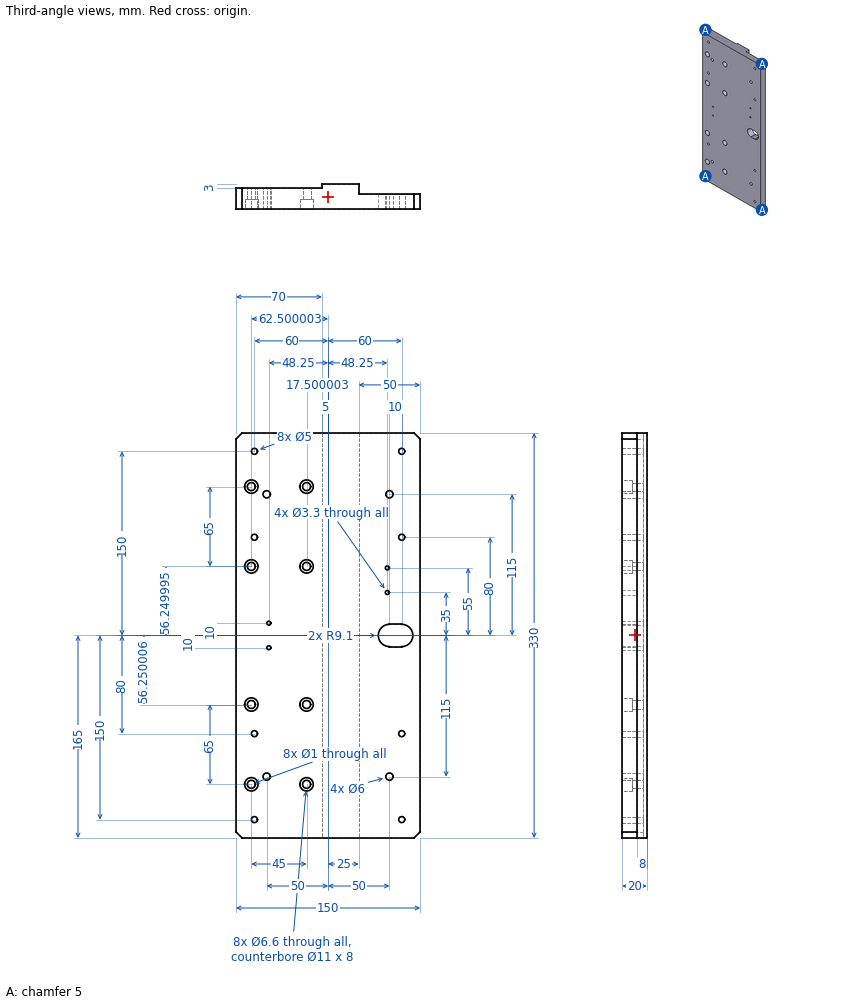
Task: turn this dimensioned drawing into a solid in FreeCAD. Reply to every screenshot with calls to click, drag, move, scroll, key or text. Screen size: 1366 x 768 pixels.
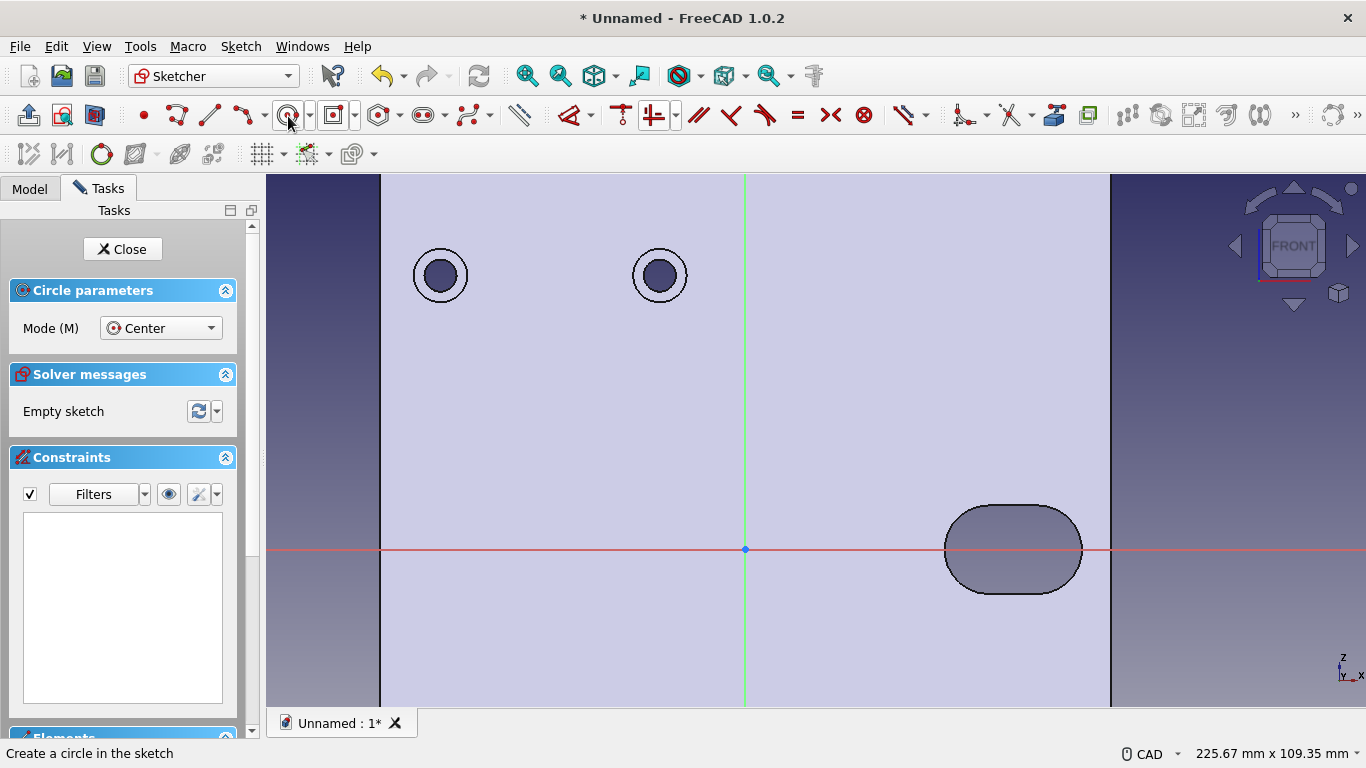
scroll(980, 379, up, 6)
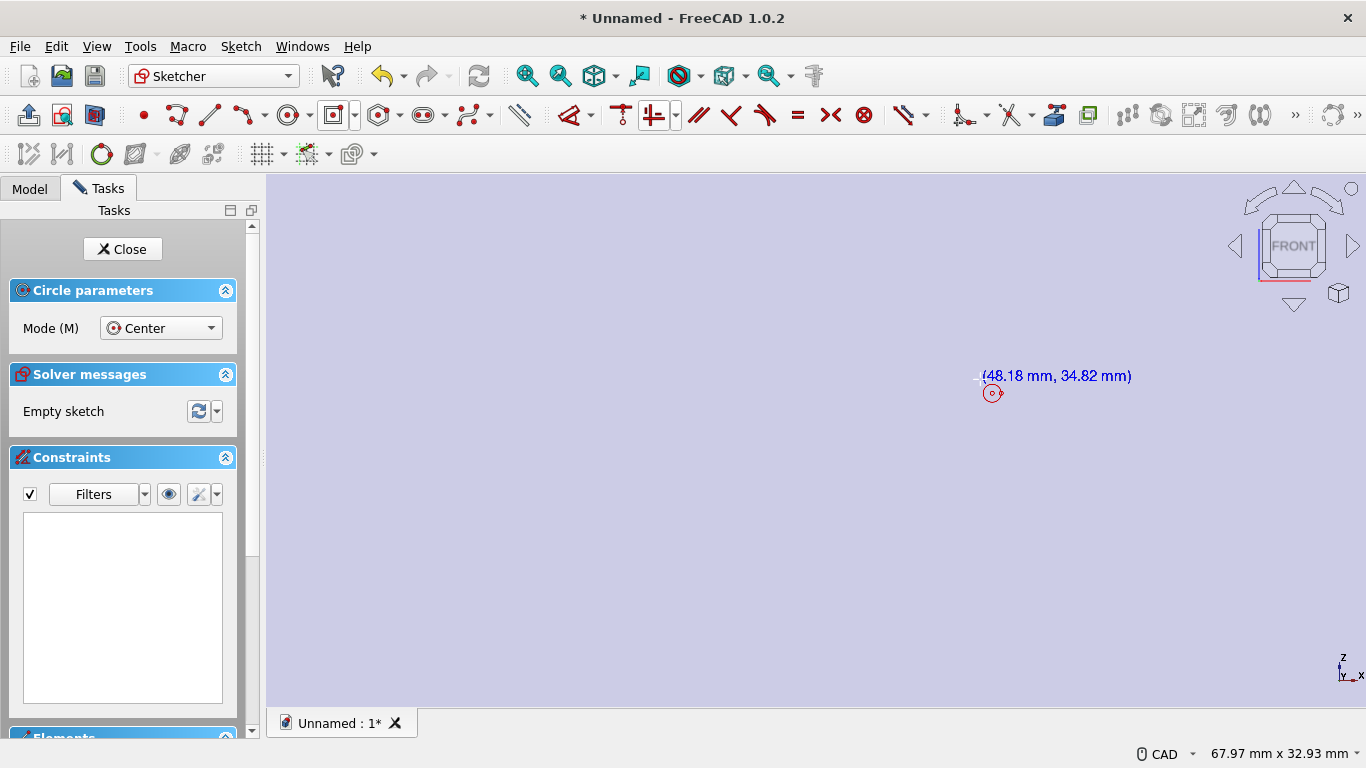
click(980, 379)
move(999, 360)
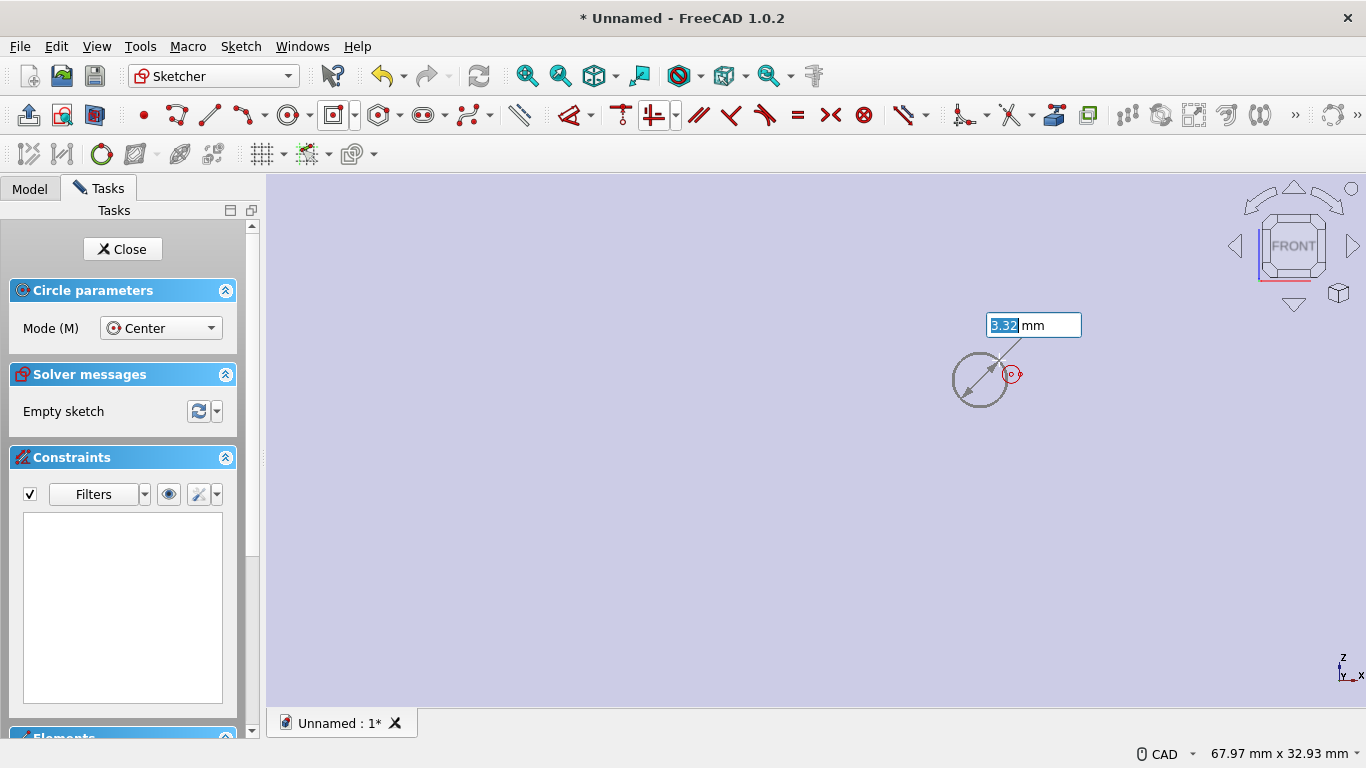
text(3.3)
key(Return)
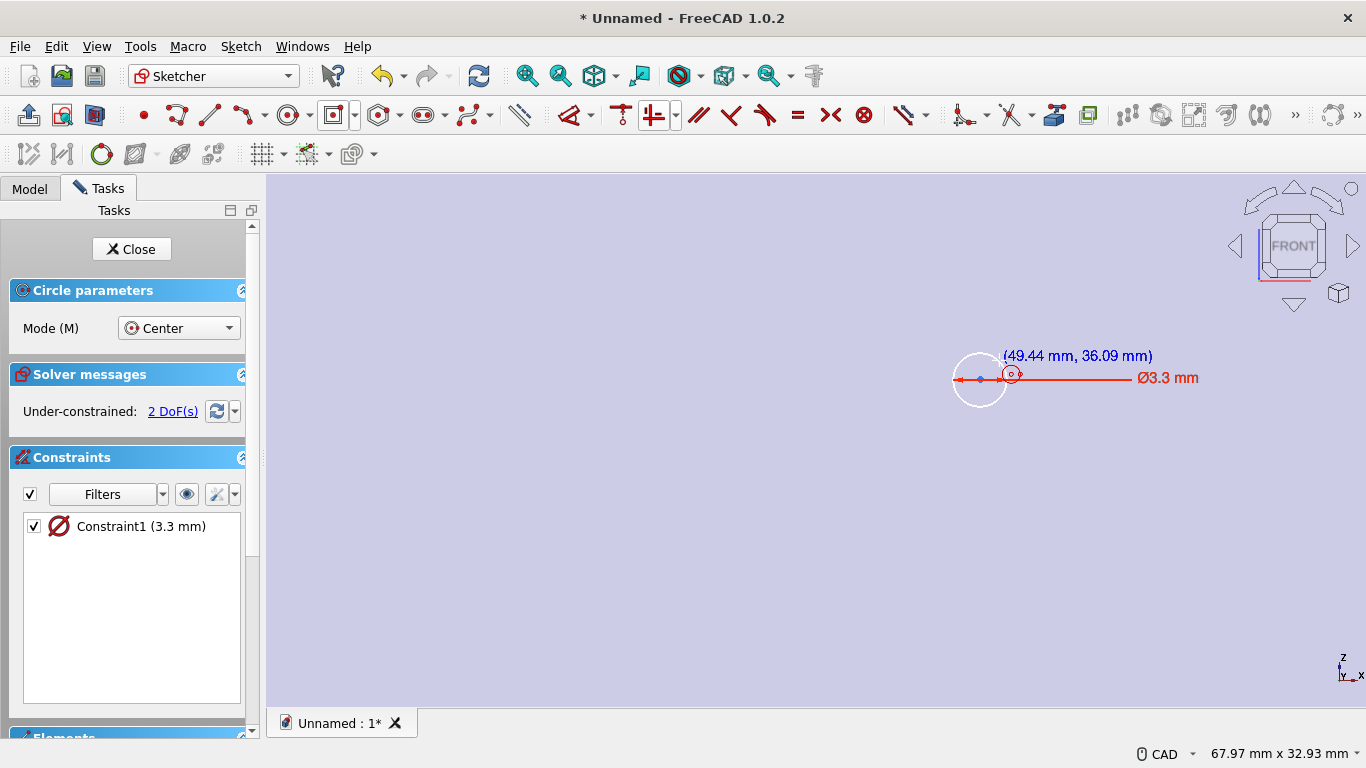
scroll(984, 380, down, 6)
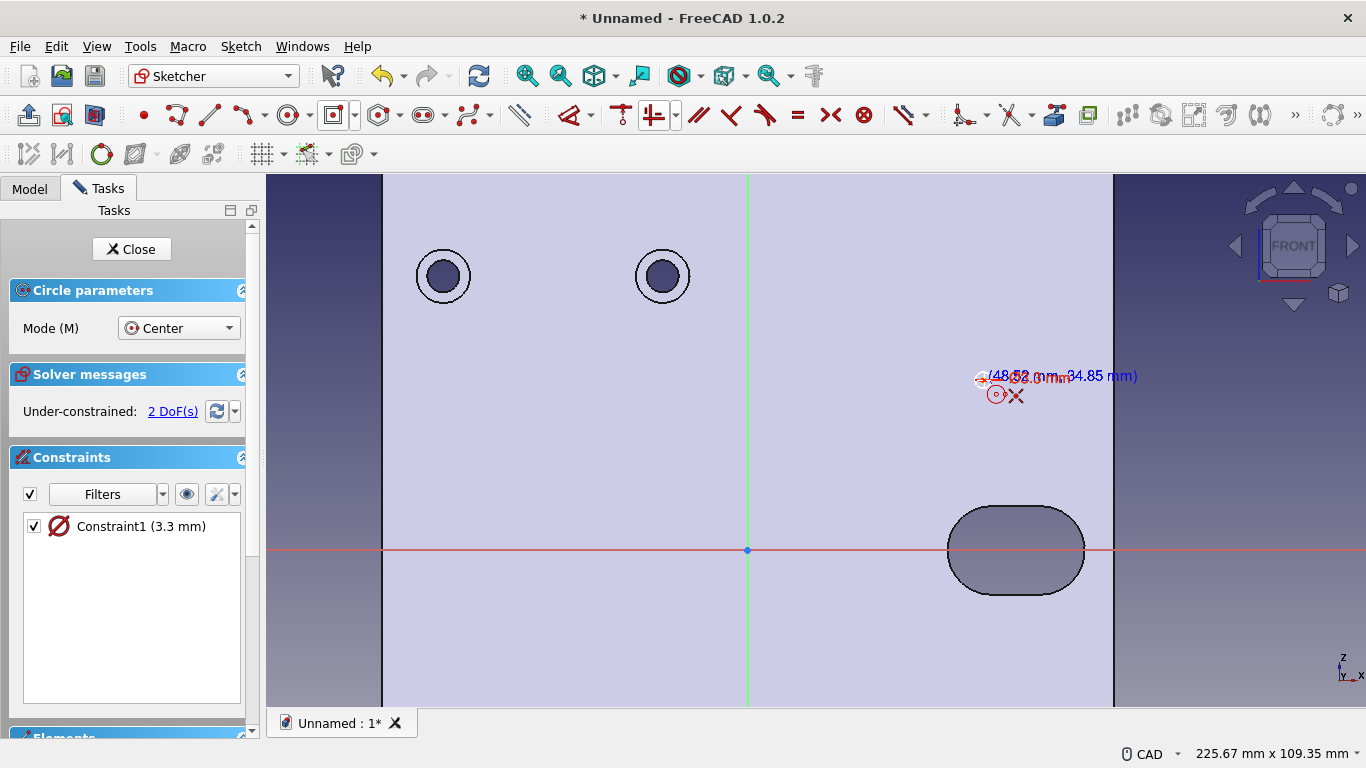
scroll(983, 282, up, 6)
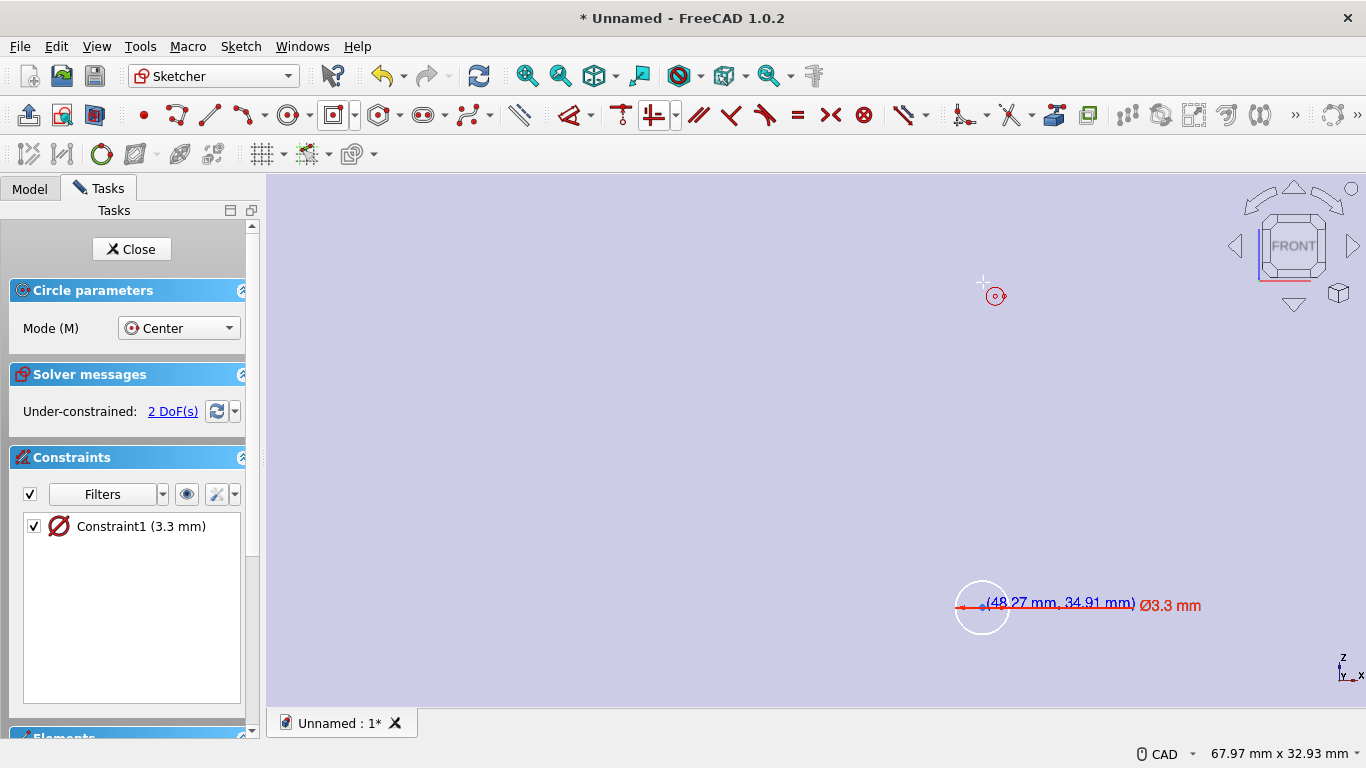
click(982, 283)
move(1001, 264)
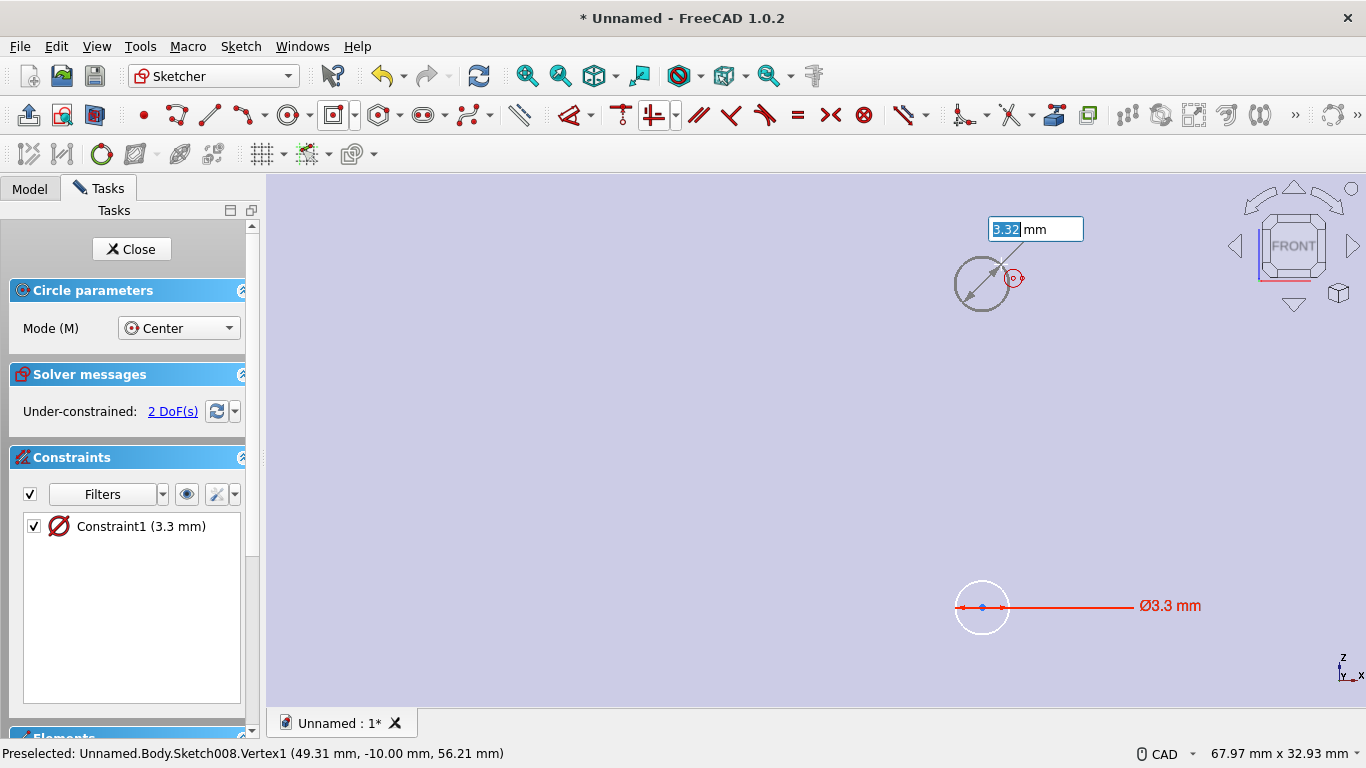
text(3.3)
key(Return)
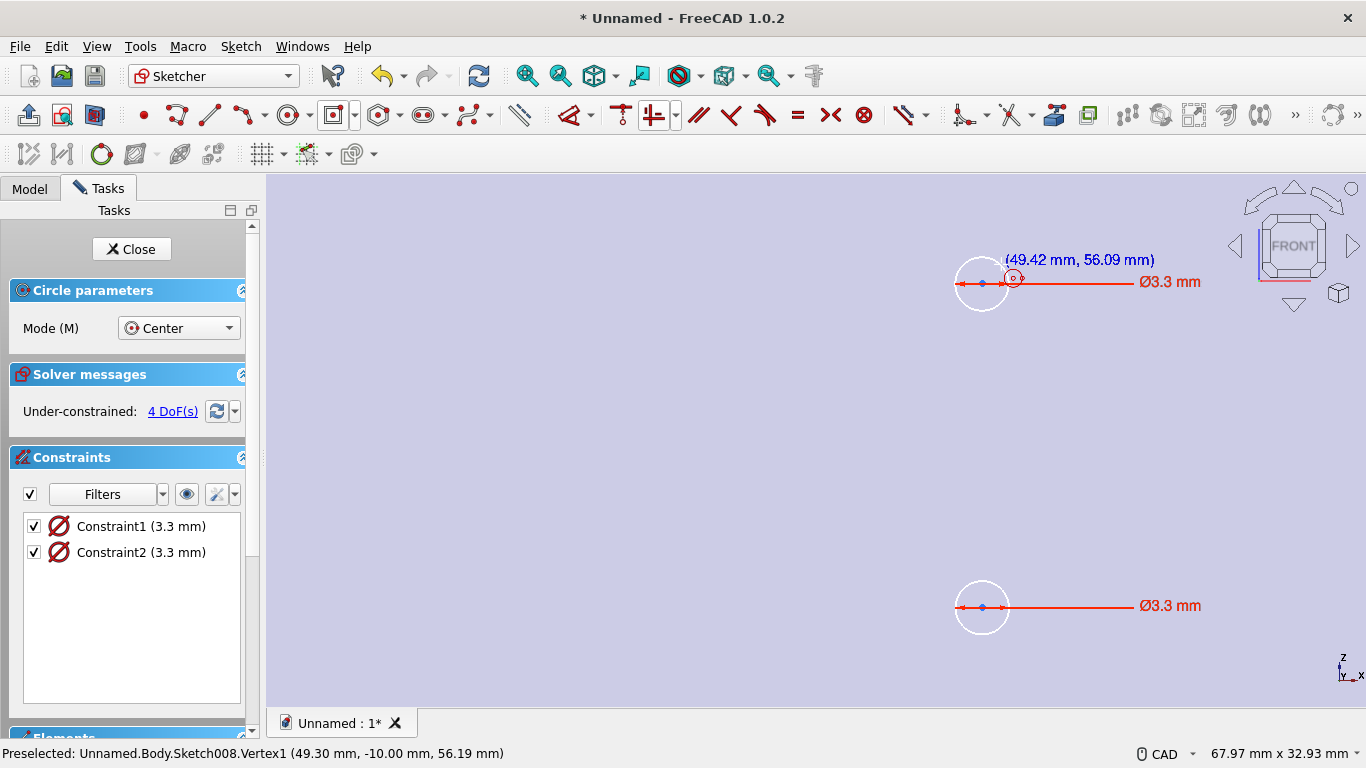
scroll(983, 282, down, 6)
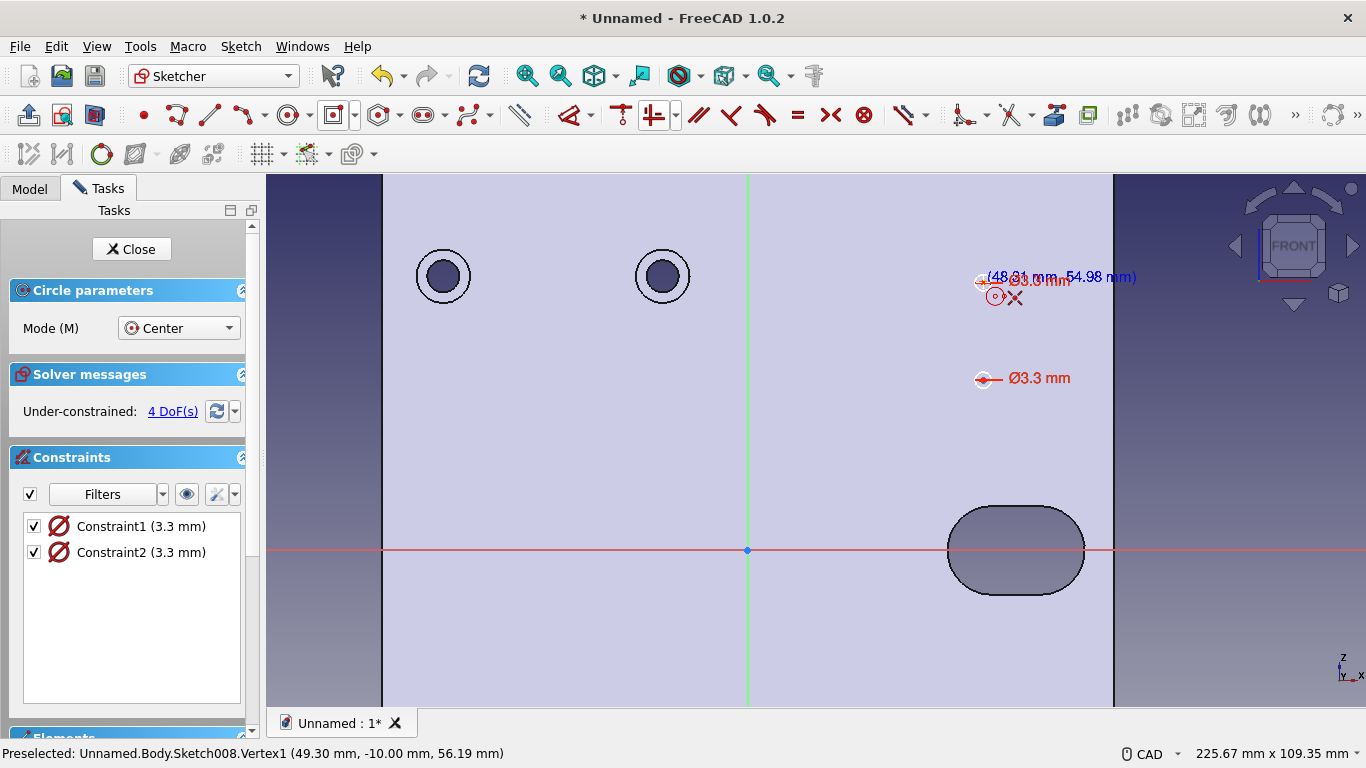
scroll(513, 502, up, 6)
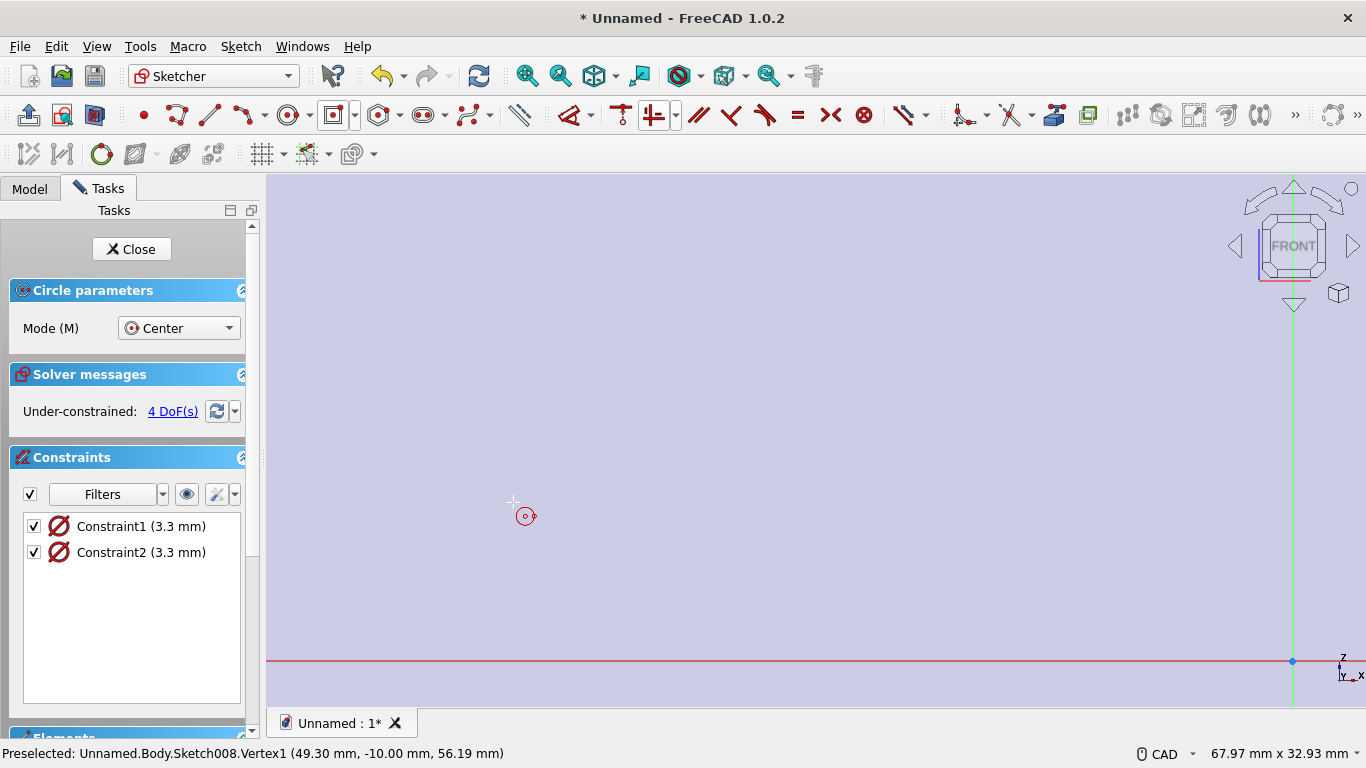
click(512, 500)
move(531, 481)